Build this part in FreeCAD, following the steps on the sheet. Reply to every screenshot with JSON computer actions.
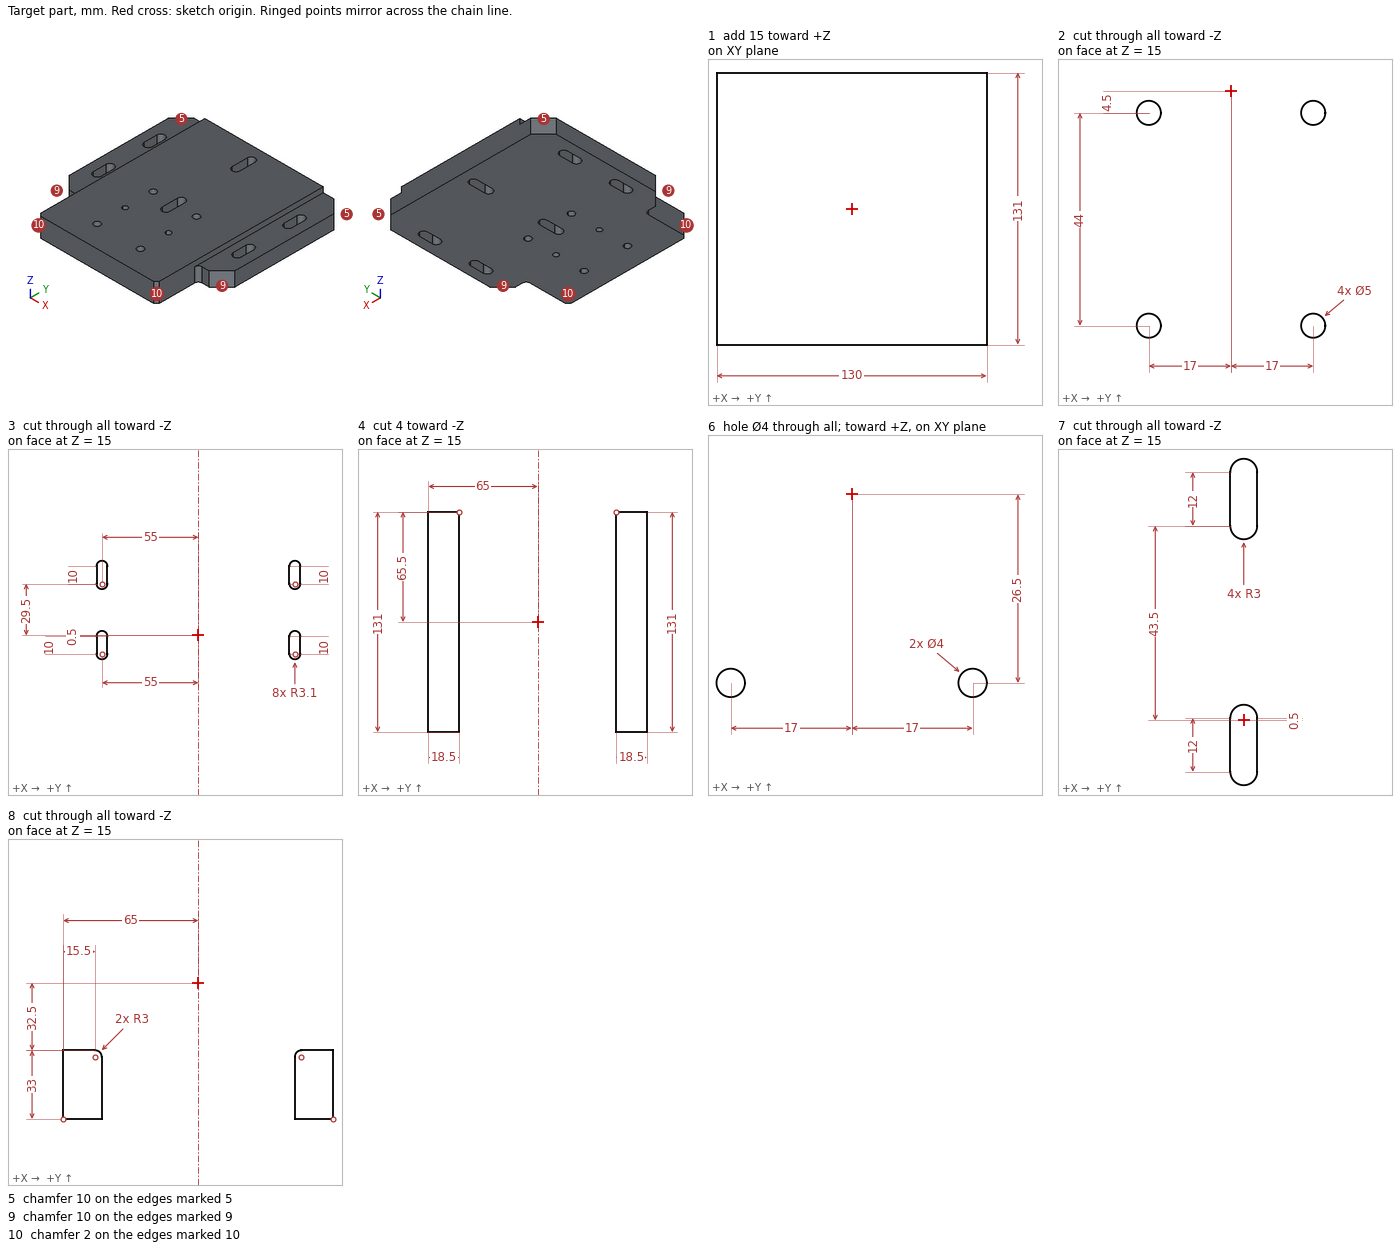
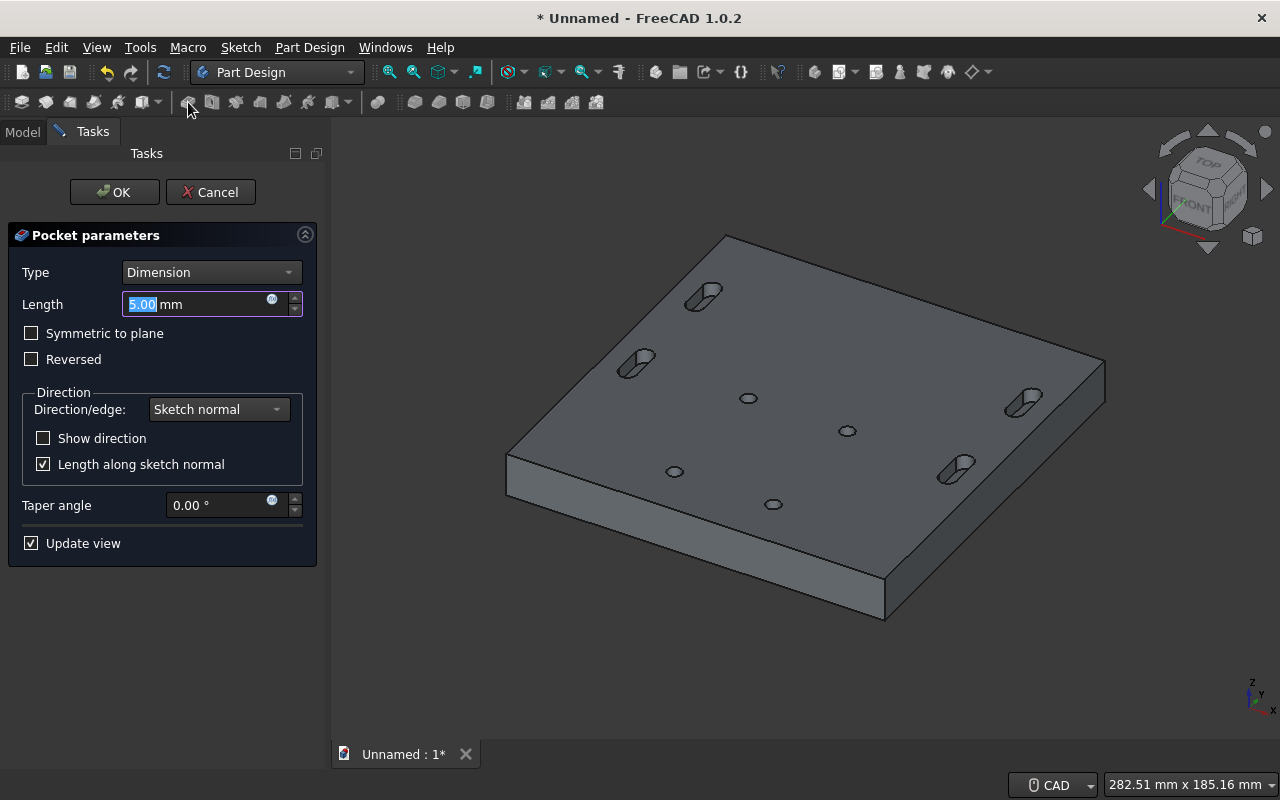
{"action": "left_click", "coordinate": [212, 272]}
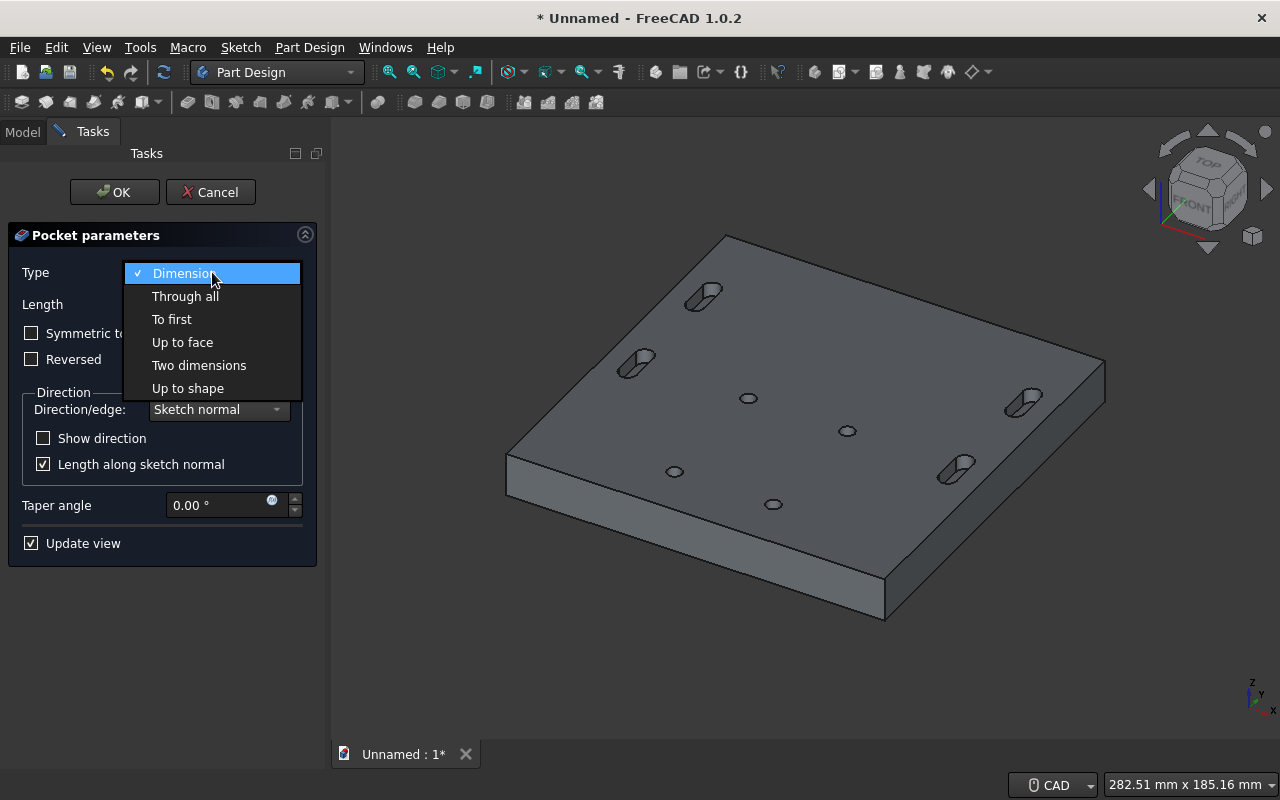
{"action": "left_click", "coordinate": [212, 296]}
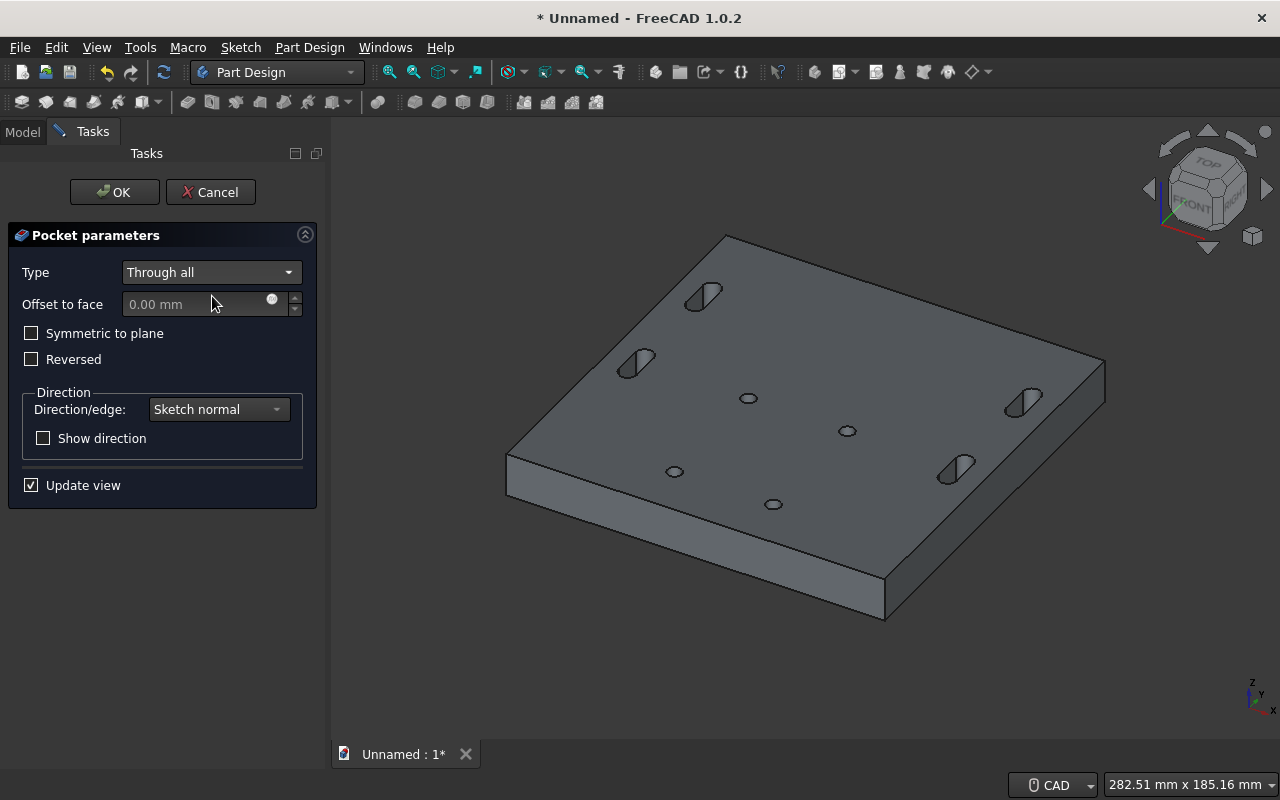
{"action": "left_click", "coordinate": [115, 192]}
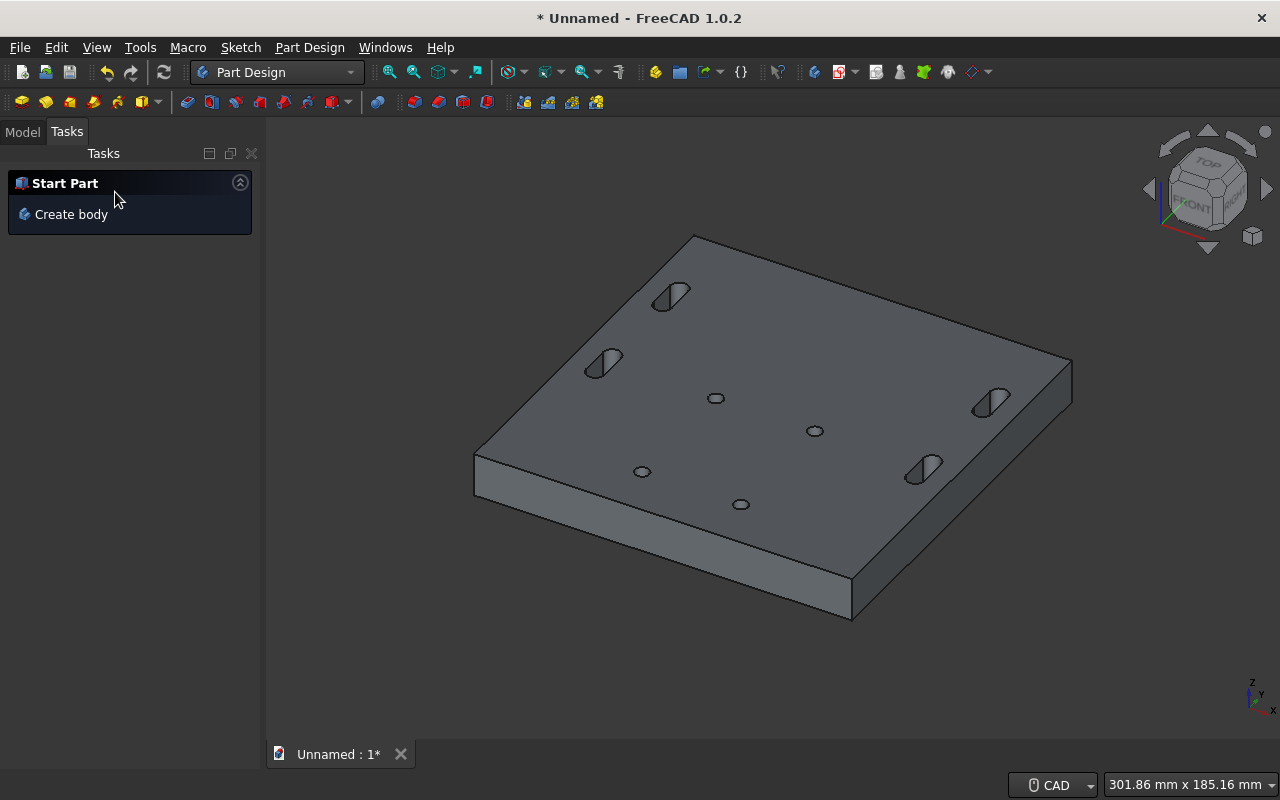
{"action": "left_click", "coordinate": [890, 362]}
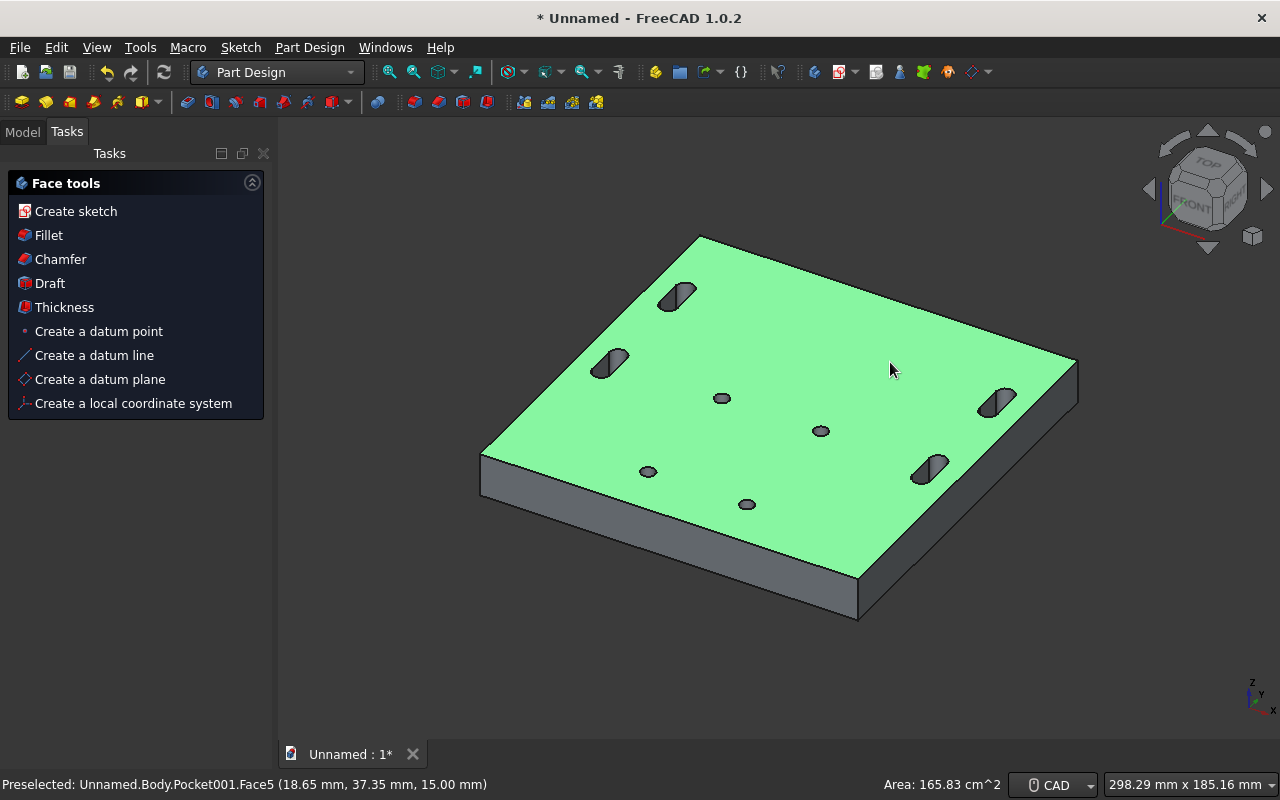
{"action": "left_click", "coordinate": [840, 72]}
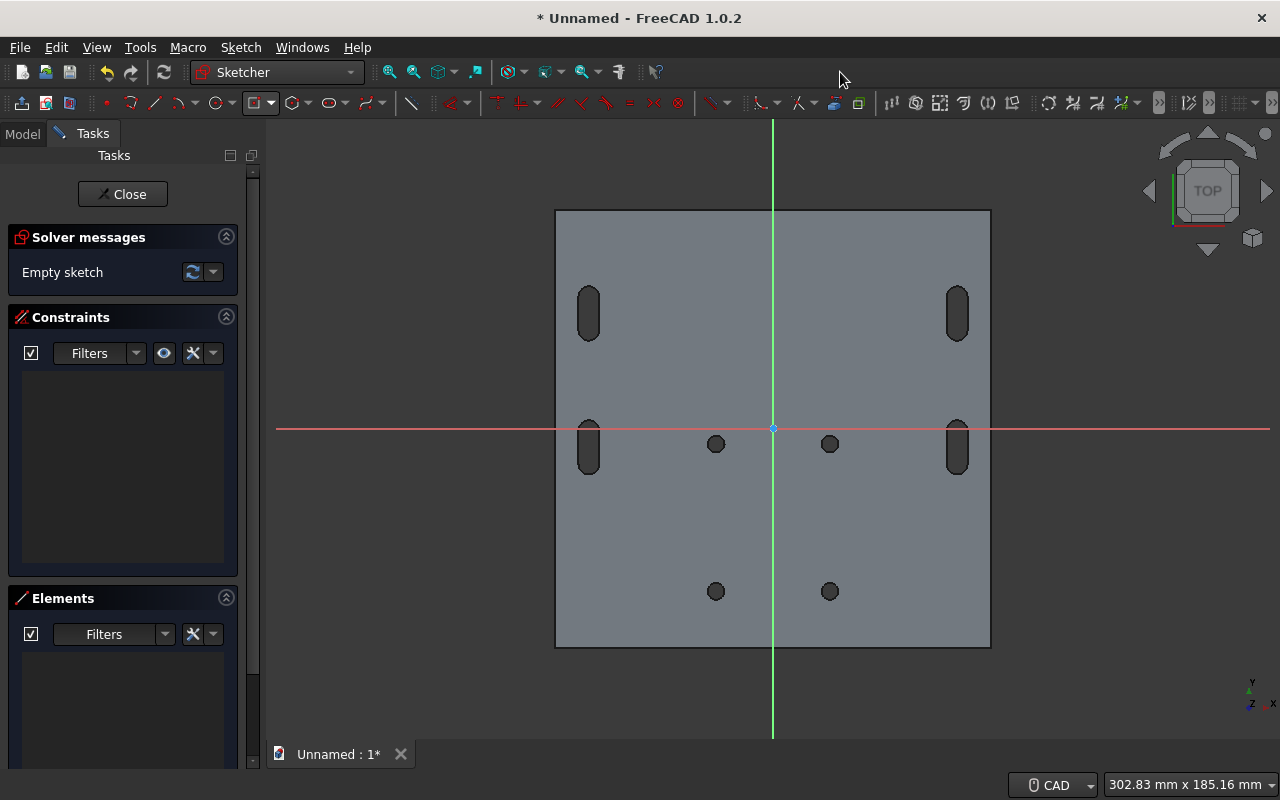
{"action": "key", "text": "g r"}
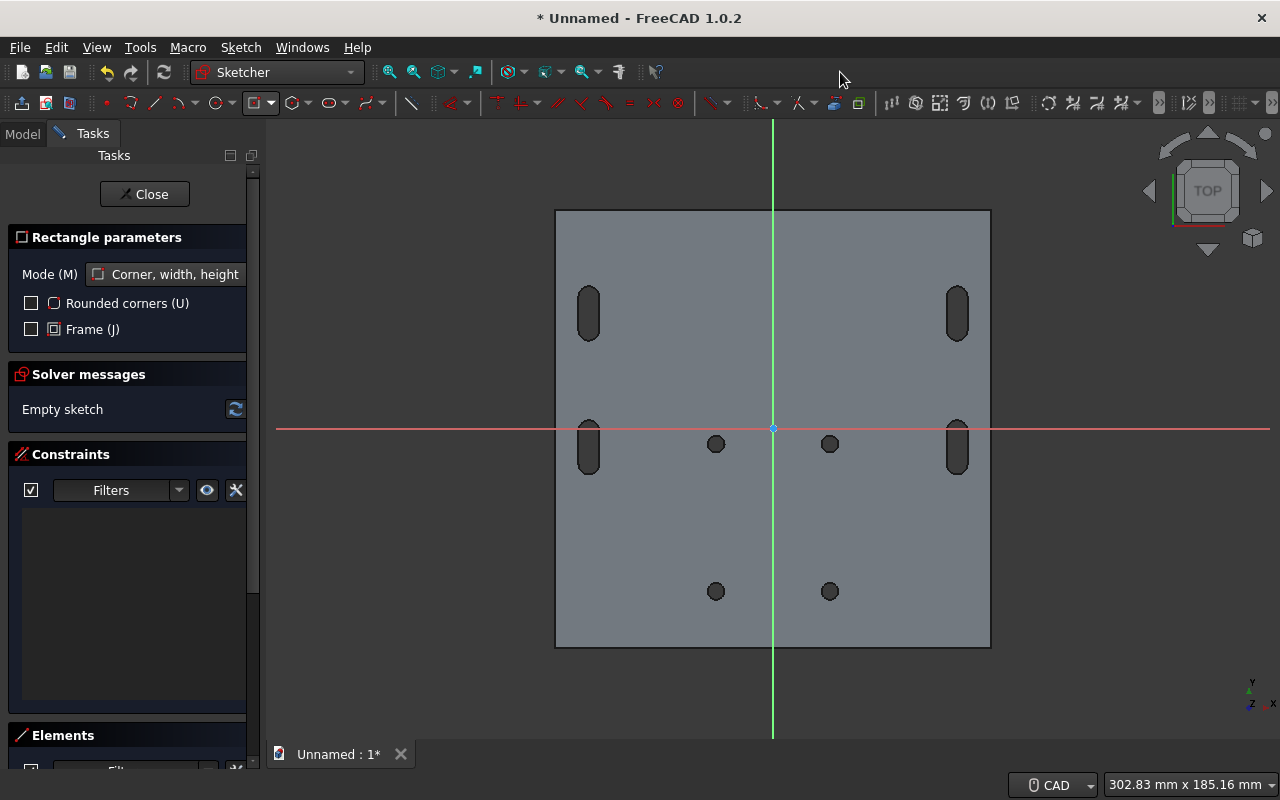
{"action": "left_click", "coordinate": [555, 210]}
{"action": "mouse_move", "coordinate": [617, 648]}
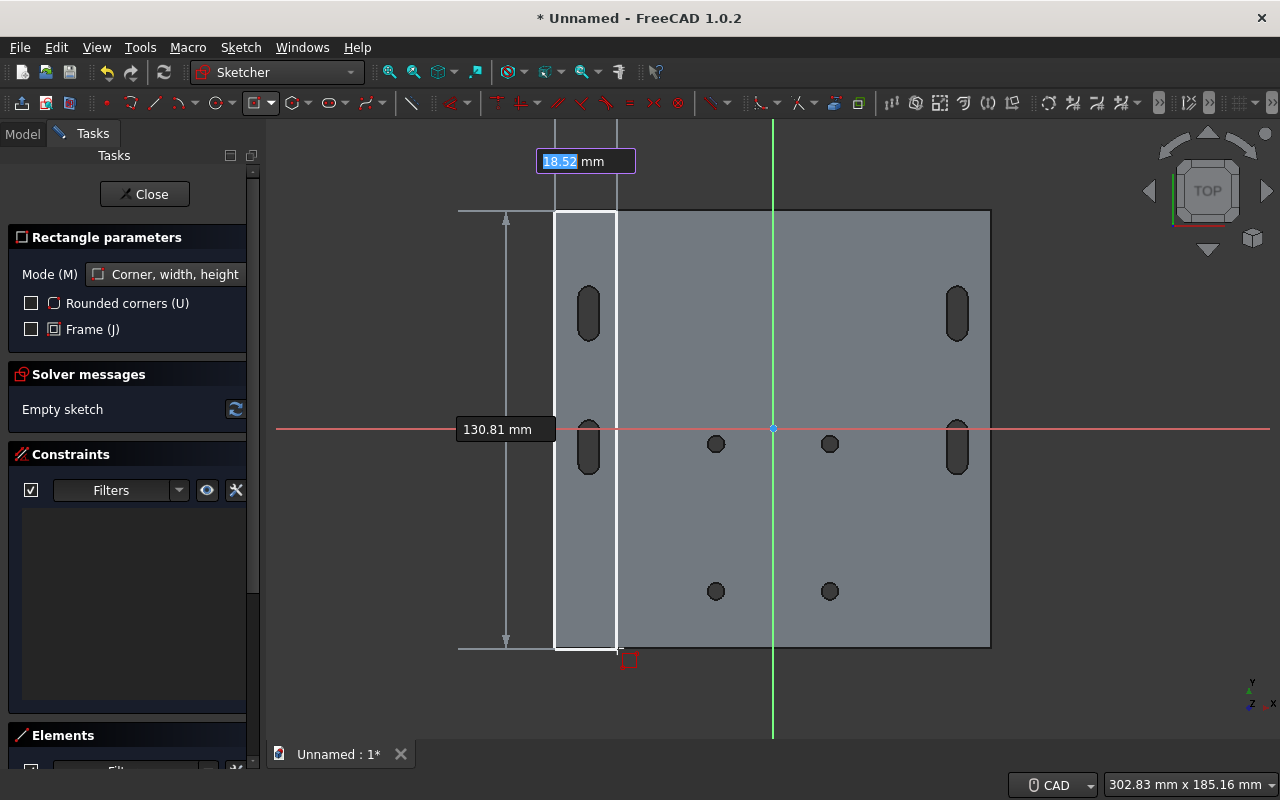
{"action": "type", "text": "18.5"}
{"action": "key", "text": "Tab"}
{"action": "type", "text": "131"}
{"action": "key", "text": "Return"}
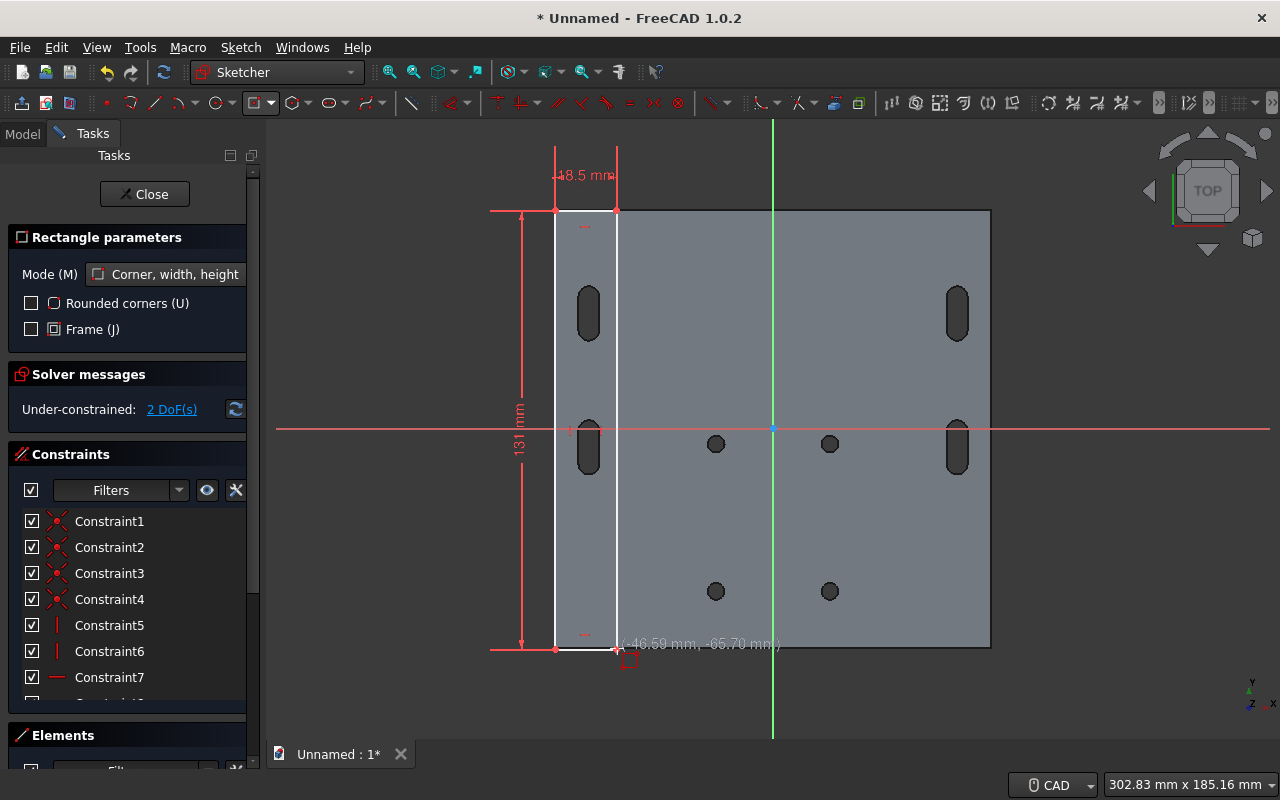
{"action": "left_click", "coordinate": [929, 210]}
{"action": "mouse_move", "coordinate": [991, 648]}